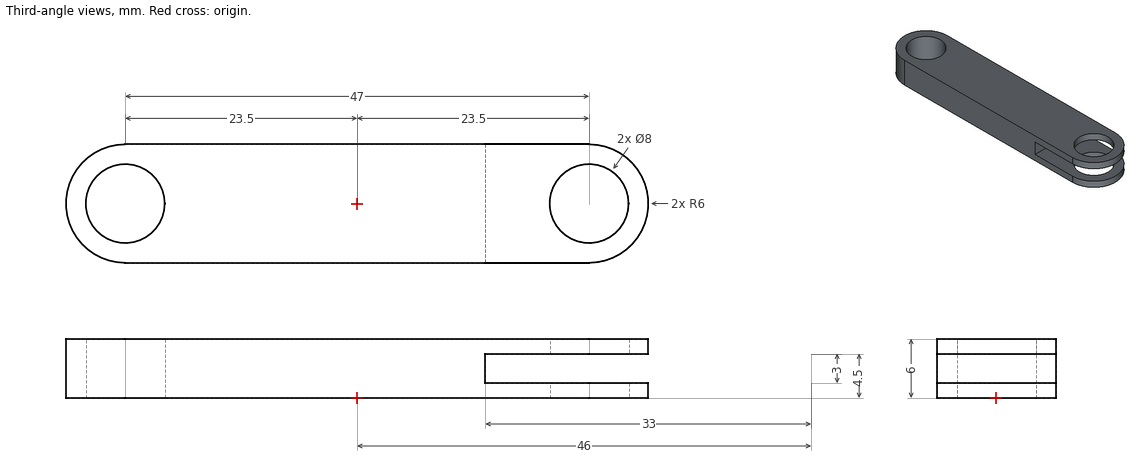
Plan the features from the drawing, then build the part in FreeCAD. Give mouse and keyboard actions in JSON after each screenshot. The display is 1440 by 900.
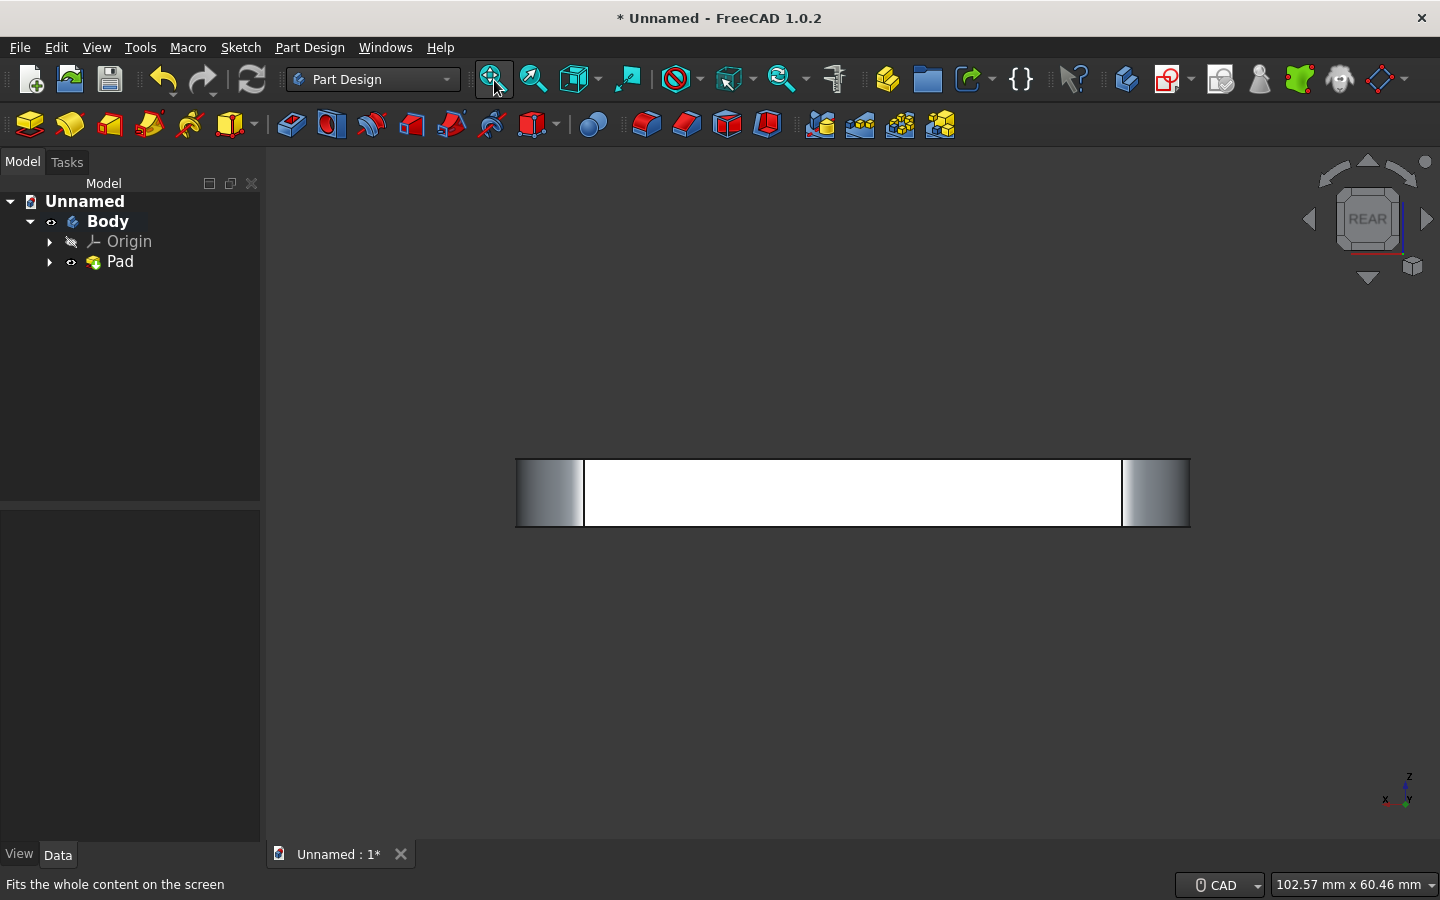
{"action": "left_click", "coordinate": [622, 492]}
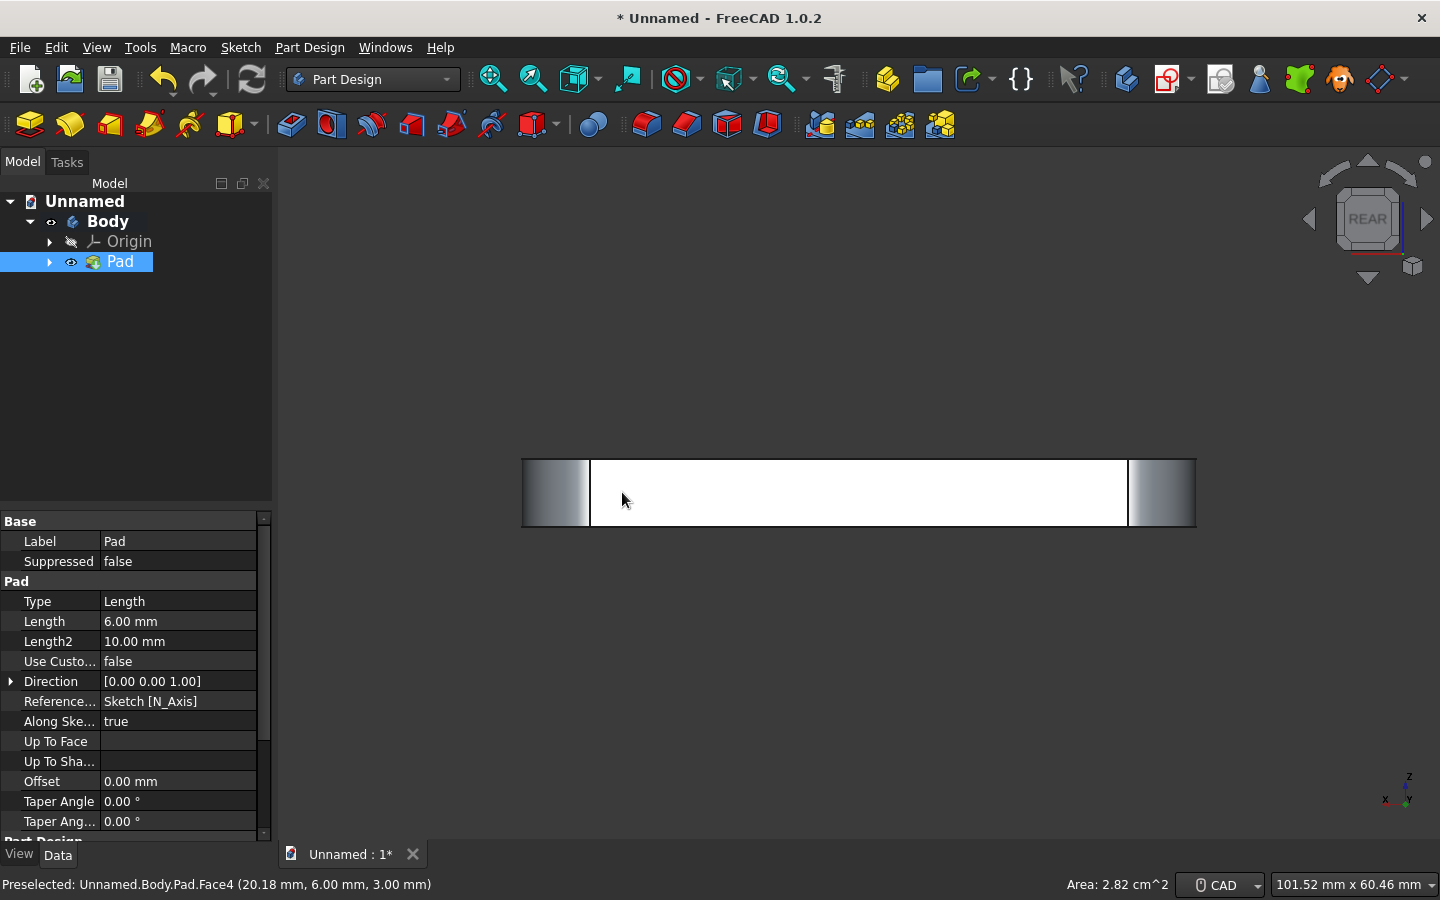
{"action": "left_click", "coordinate": [1168, 80]}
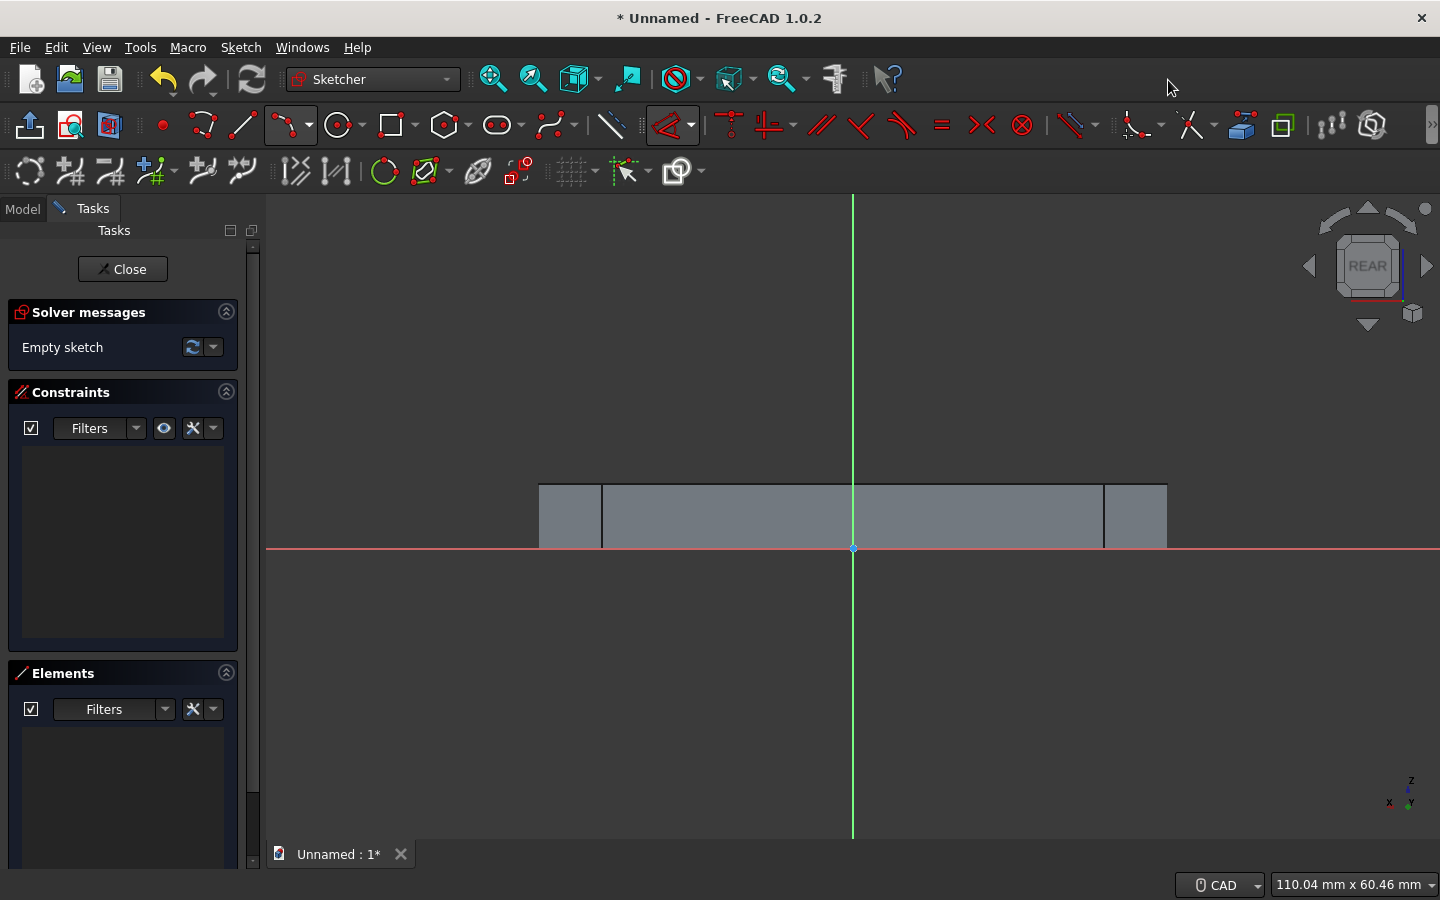
{"action": "scroll", "coordinate": [294, 541], "scroll_direction": "up", "scroll_amount": 2}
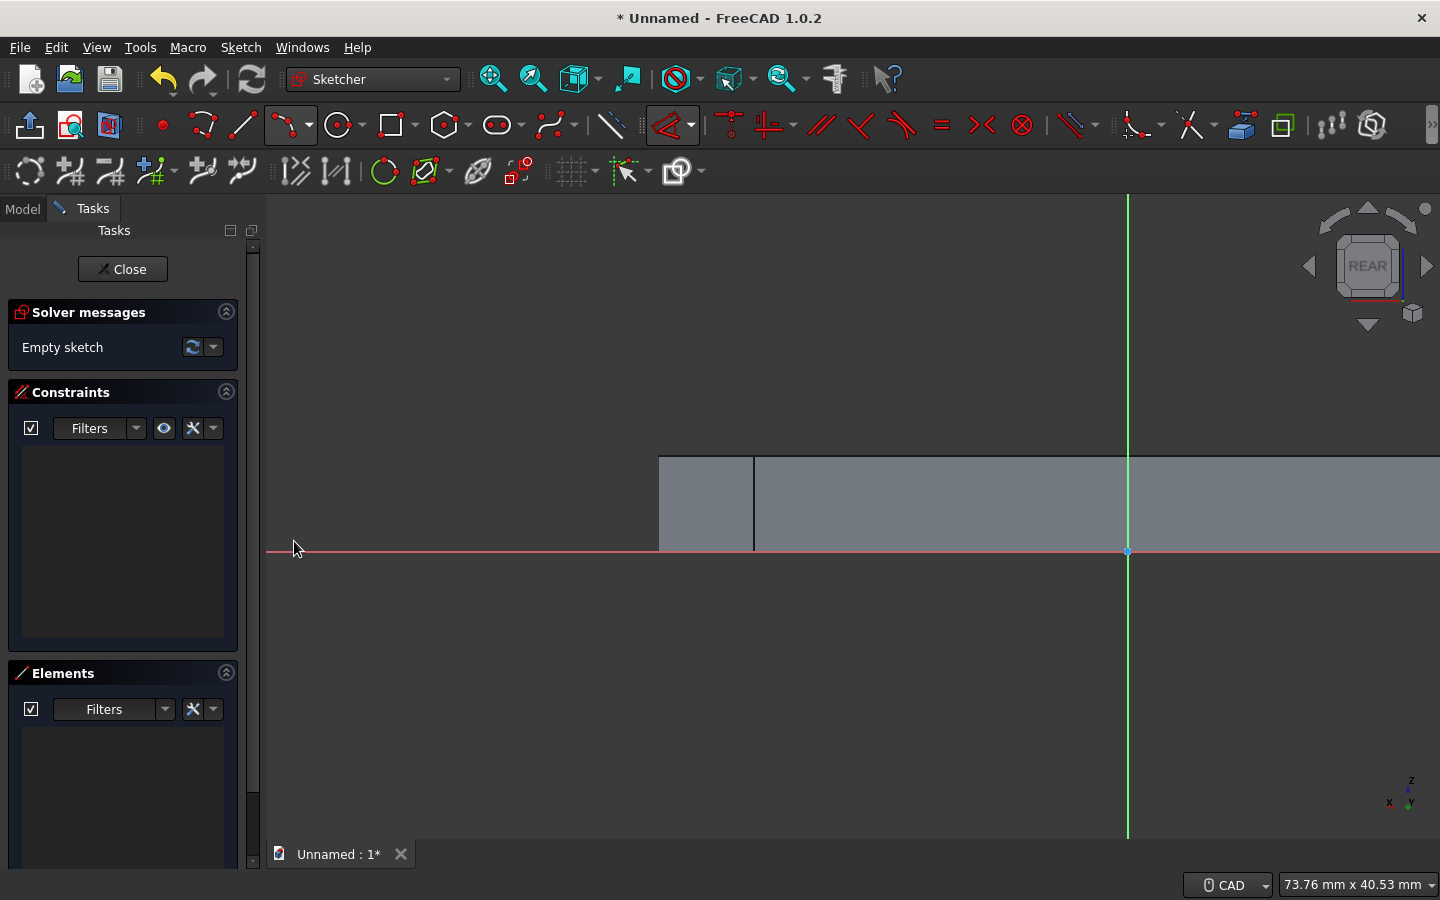
{"action": "key", "text": "g r"}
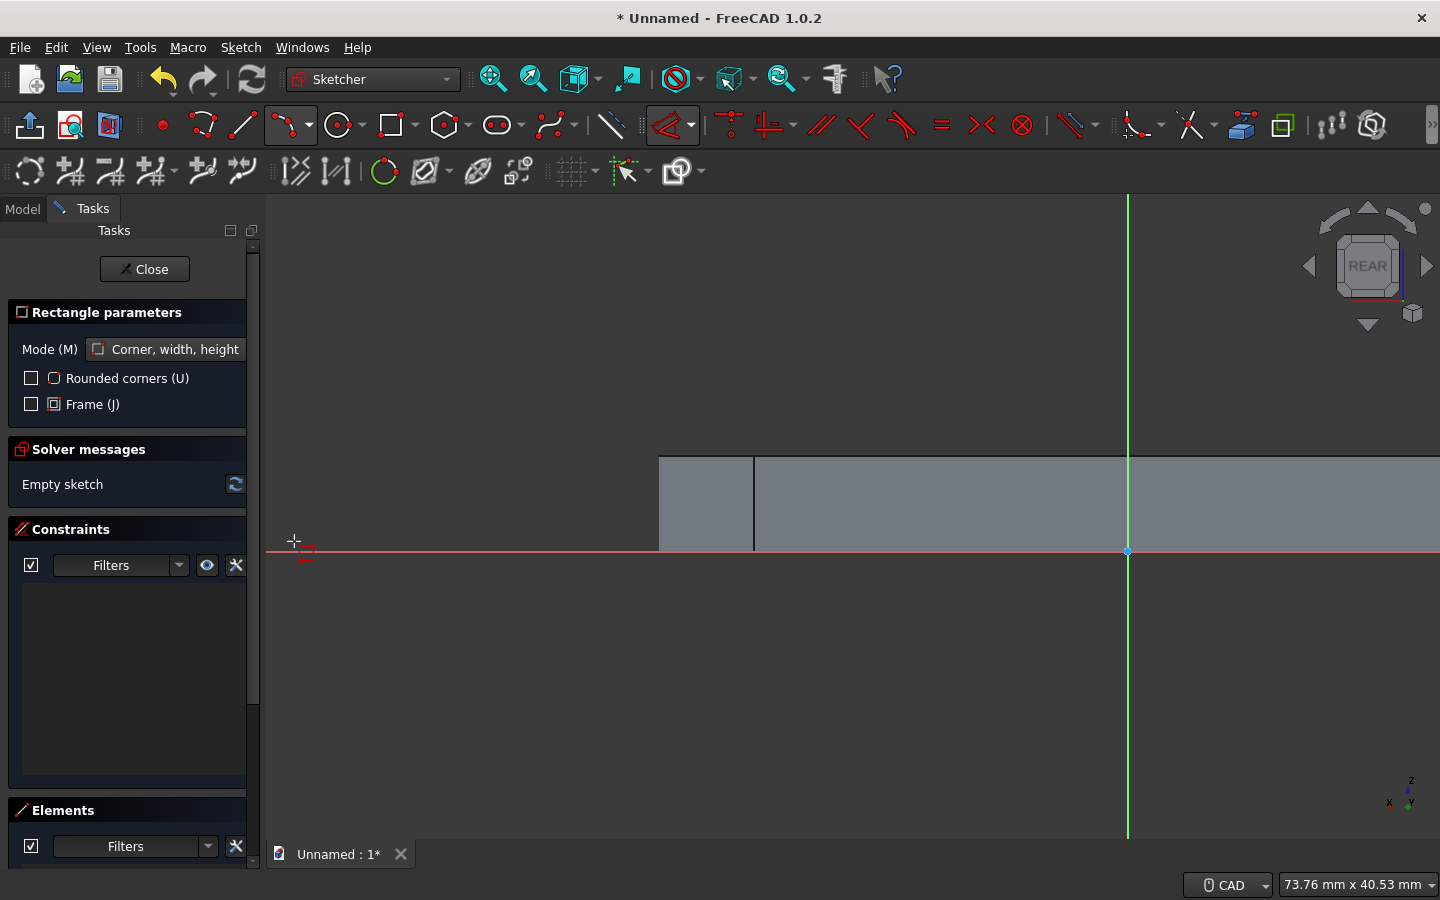
{"action": "left_click", "coordinate": [396, 480]}
{"action": "left_click", "coordinate": [921, 528]}
{"action": "key", "text": "Escape"}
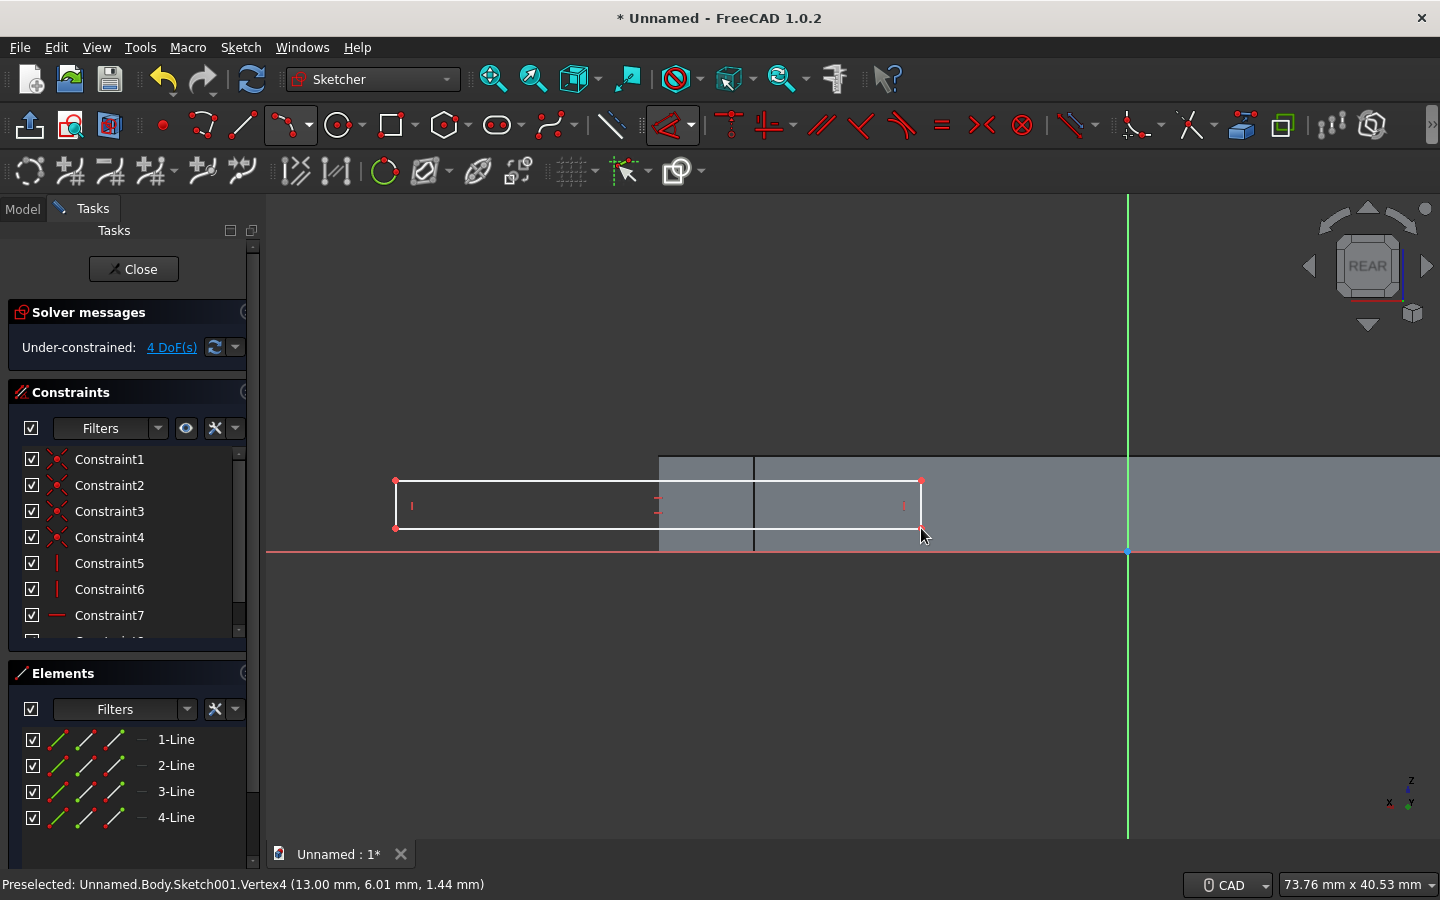
{"action": "left_click", "coordinate": [396, 495]}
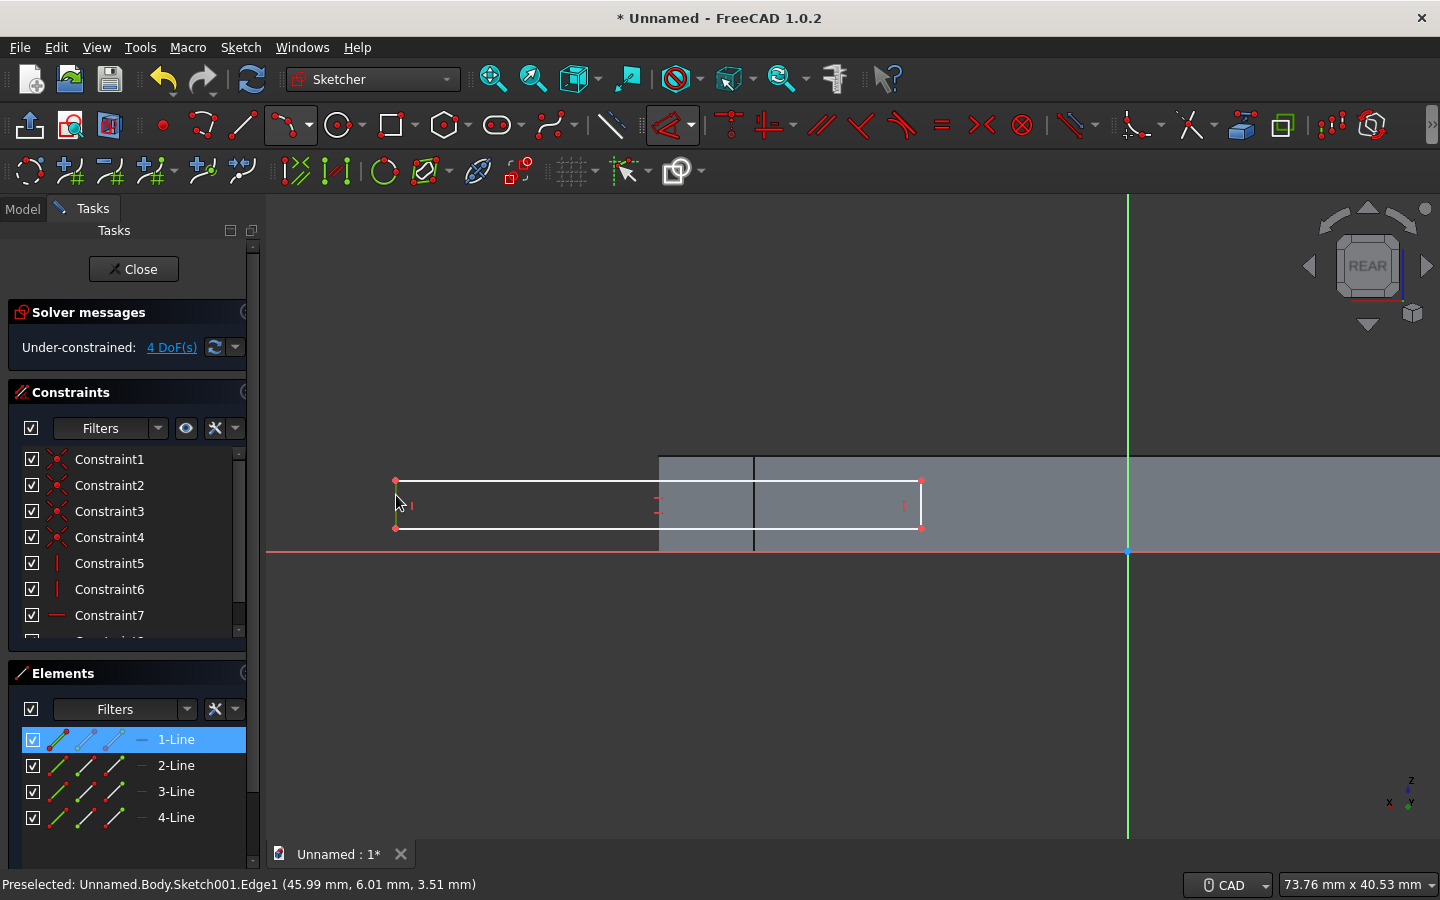
{"action": "key", "text": "i"}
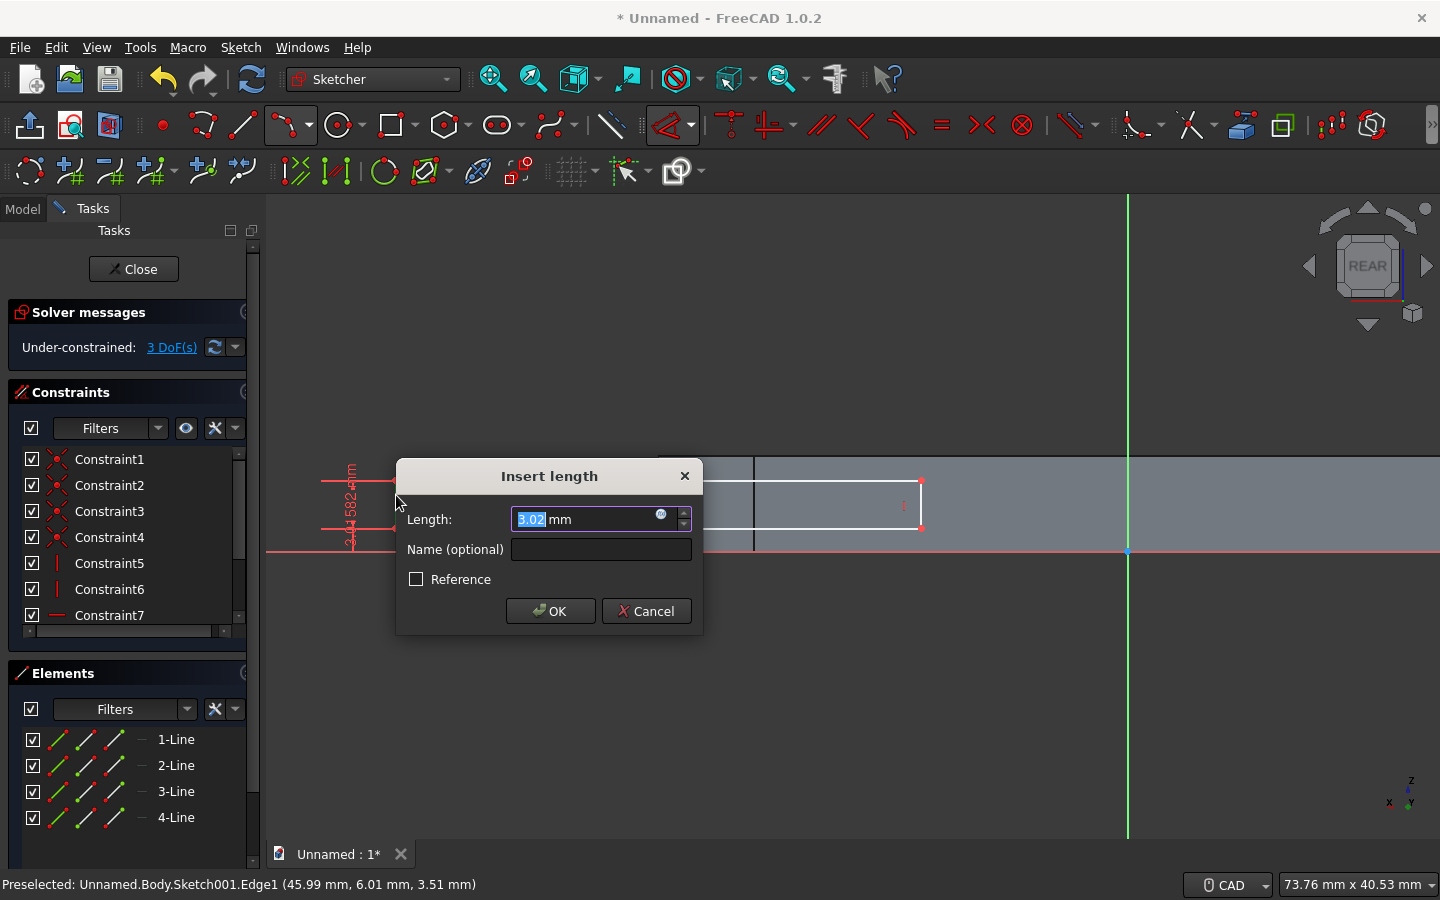
{"action": "type", "text": "3"}
{"action": "key", "text": "Return"}